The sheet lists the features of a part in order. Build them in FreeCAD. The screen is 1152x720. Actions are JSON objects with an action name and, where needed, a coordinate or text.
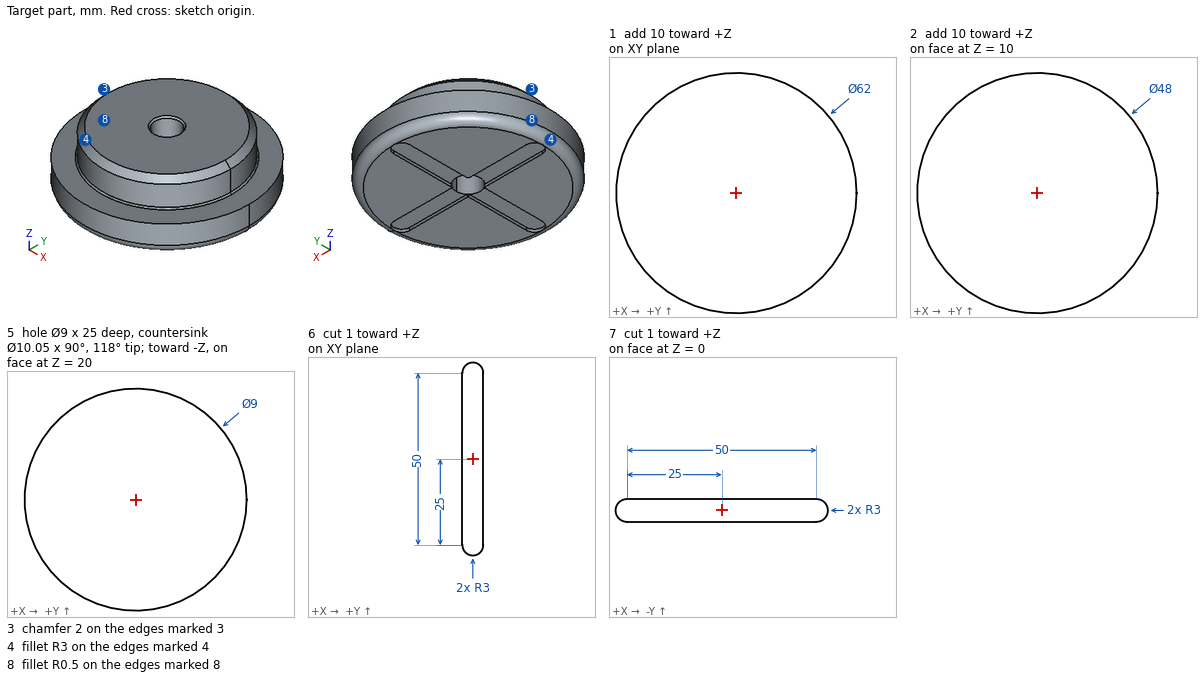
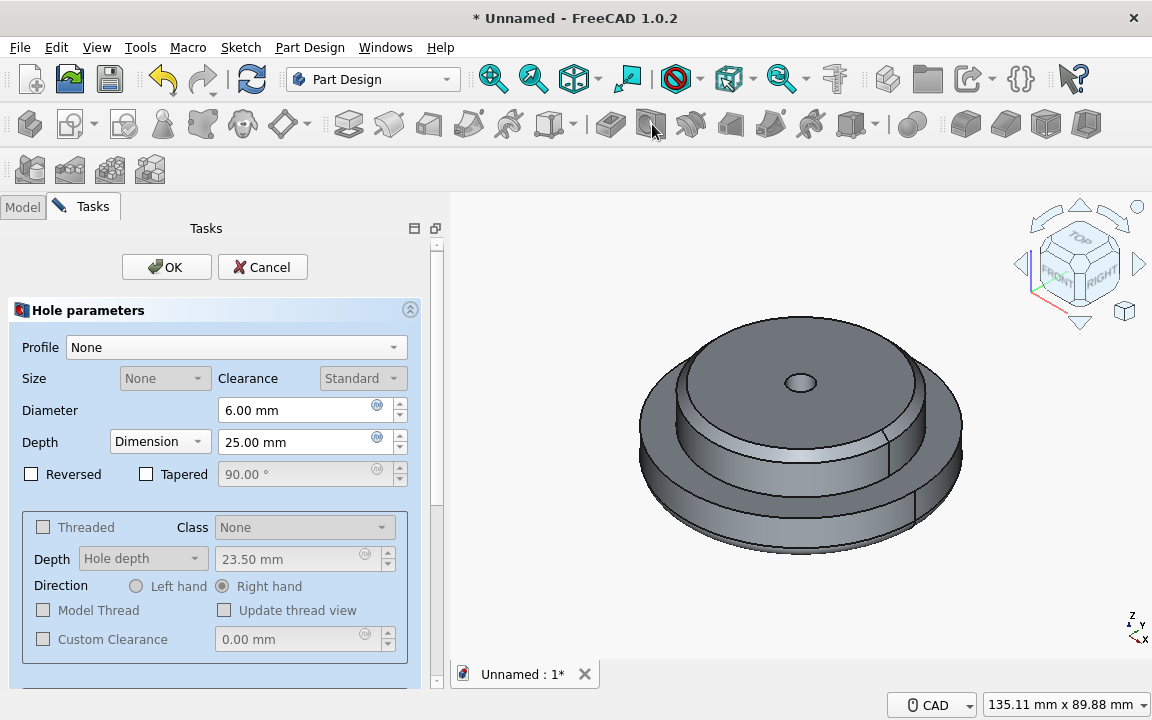
{"action": "triple_click", "coordinate": [305, 410]}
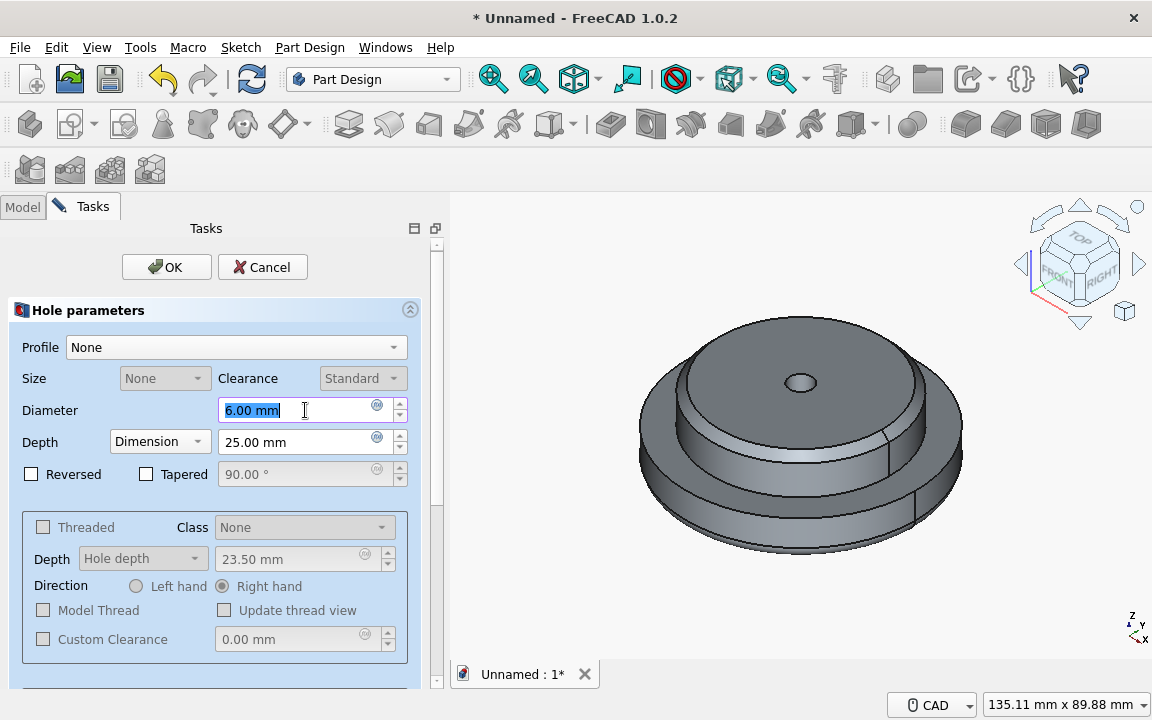
{"action": "type", "text": "9"}
{"action": "key", "text": "Tab"}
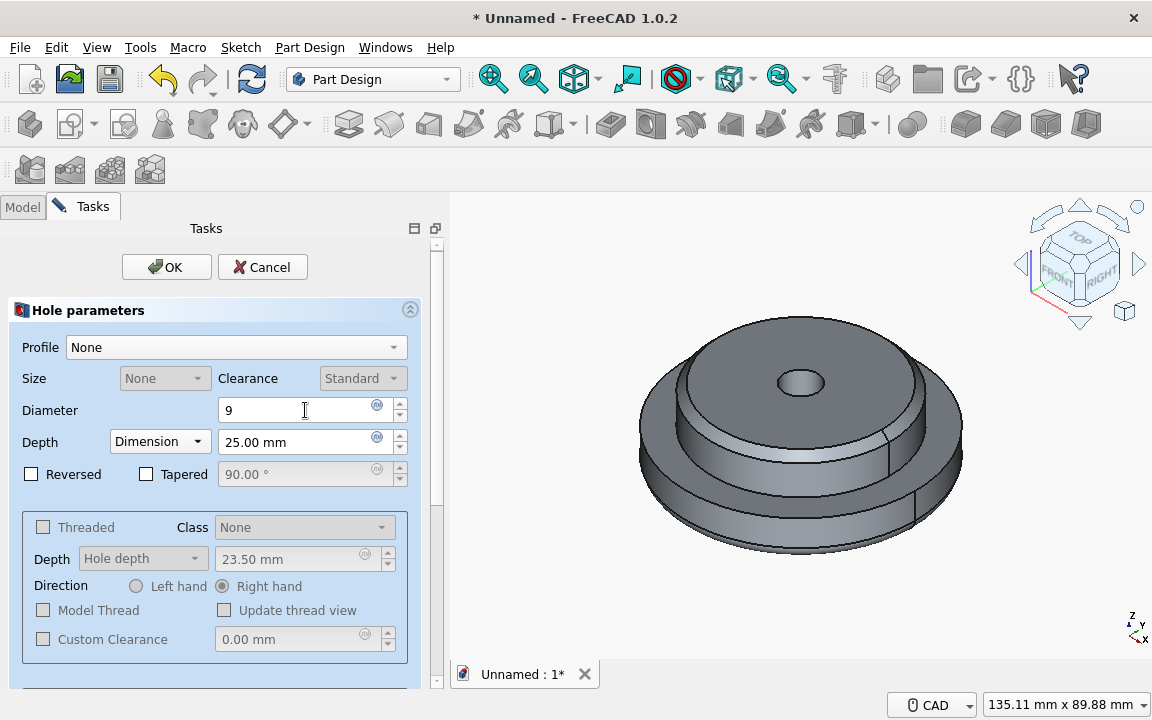
{"action": "triple_click", "coordinate": [305, 442]}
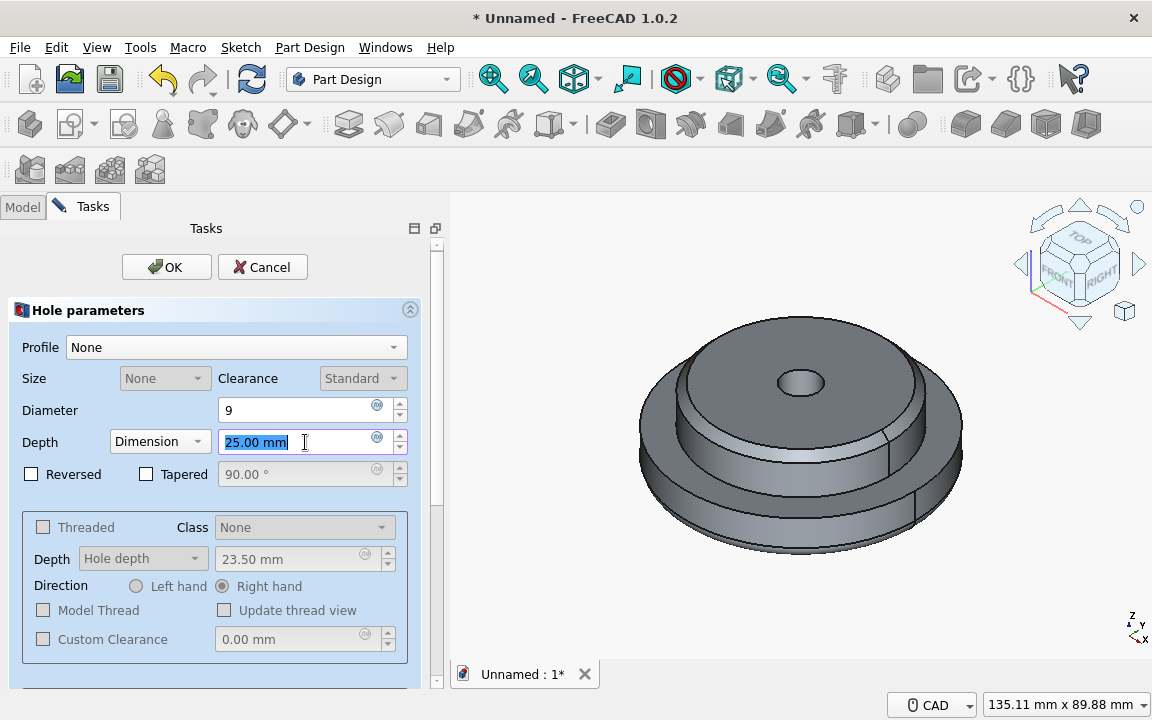
{"action": "type", "text": "25"}
{"action": "key", "text": "Tab"}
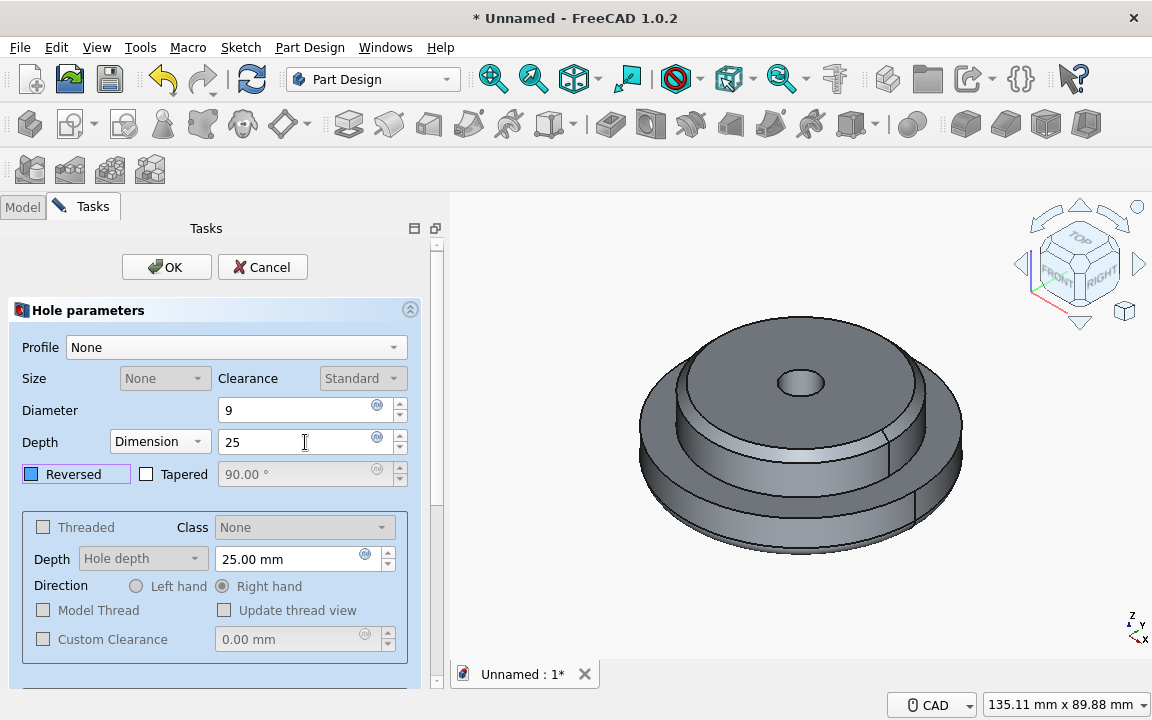
{"action": "scroll", "coordinate": [437, 463], "scroll_direction": "down", "scroll_amount": 2}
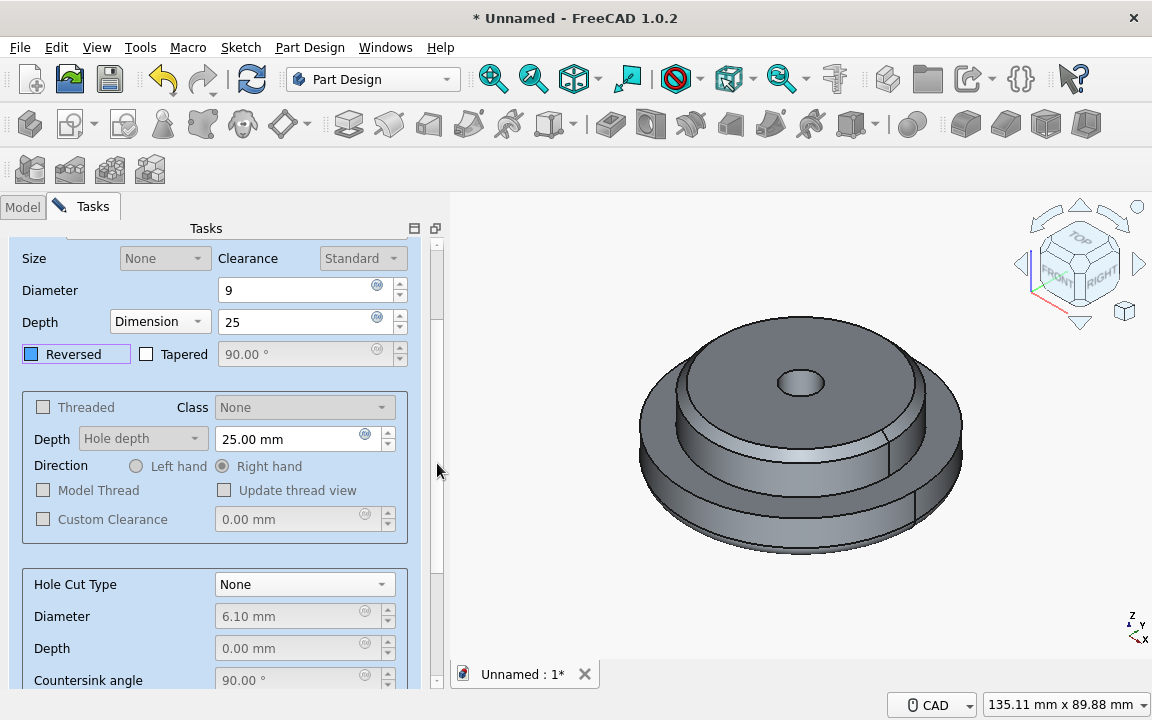
{"action": "left_click", "coordinate": [306, 584]}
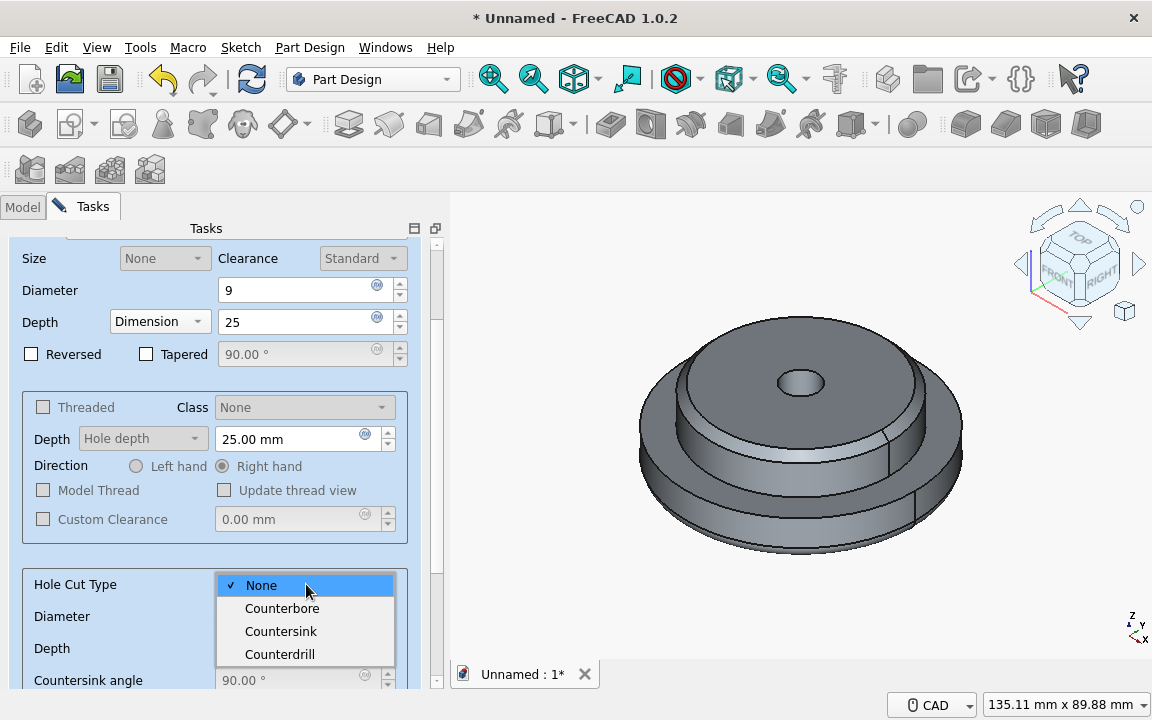
{"action": "left_click", "coordinate": [304, 632]}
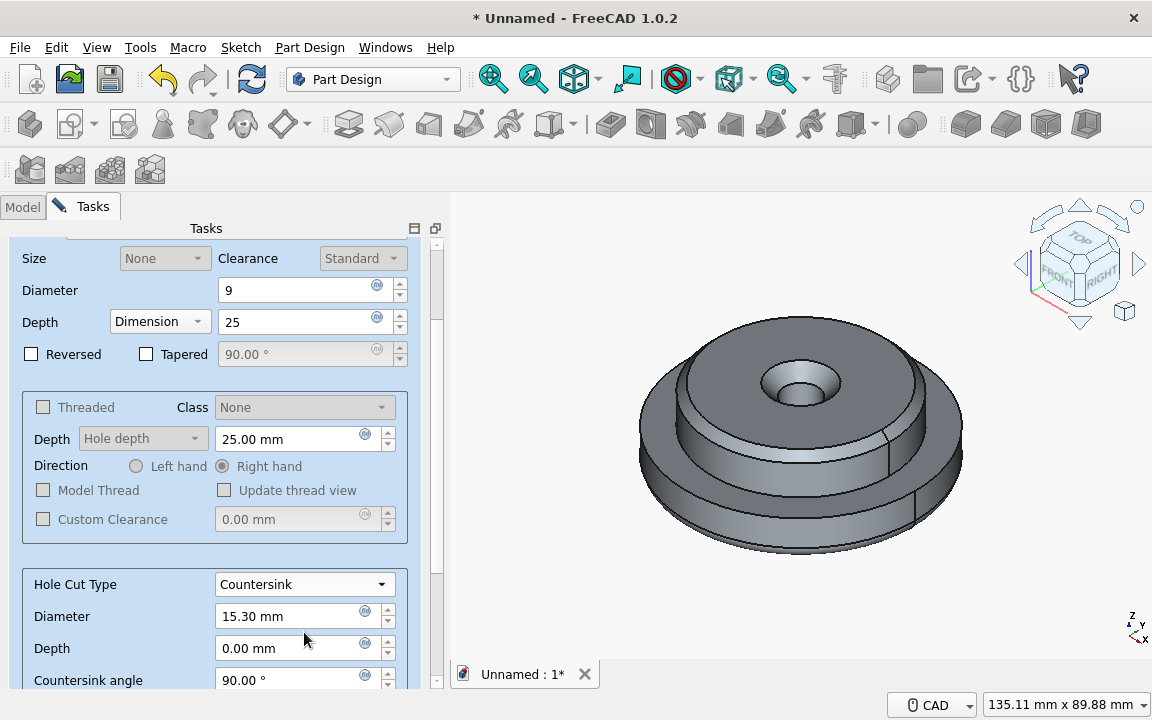
{"action": "triple_click", "coordinate": [298, 616]}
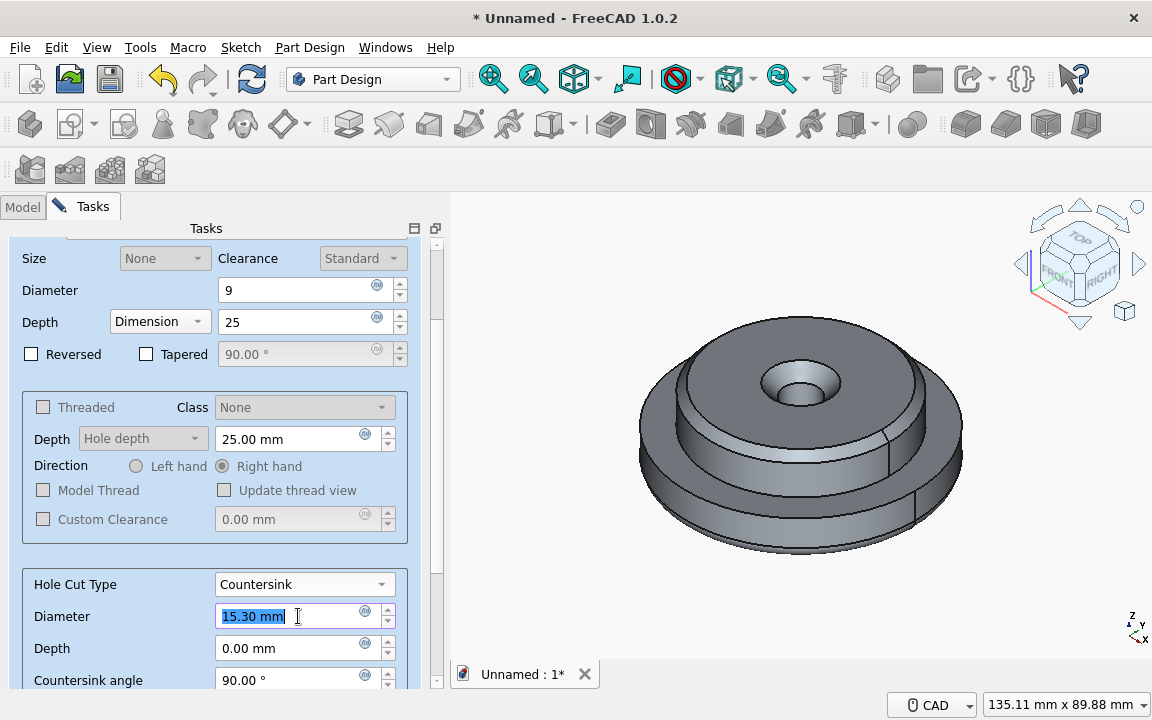
{"action": "type", "text": "10.05"}
{"action": "key", "text": "Tab"}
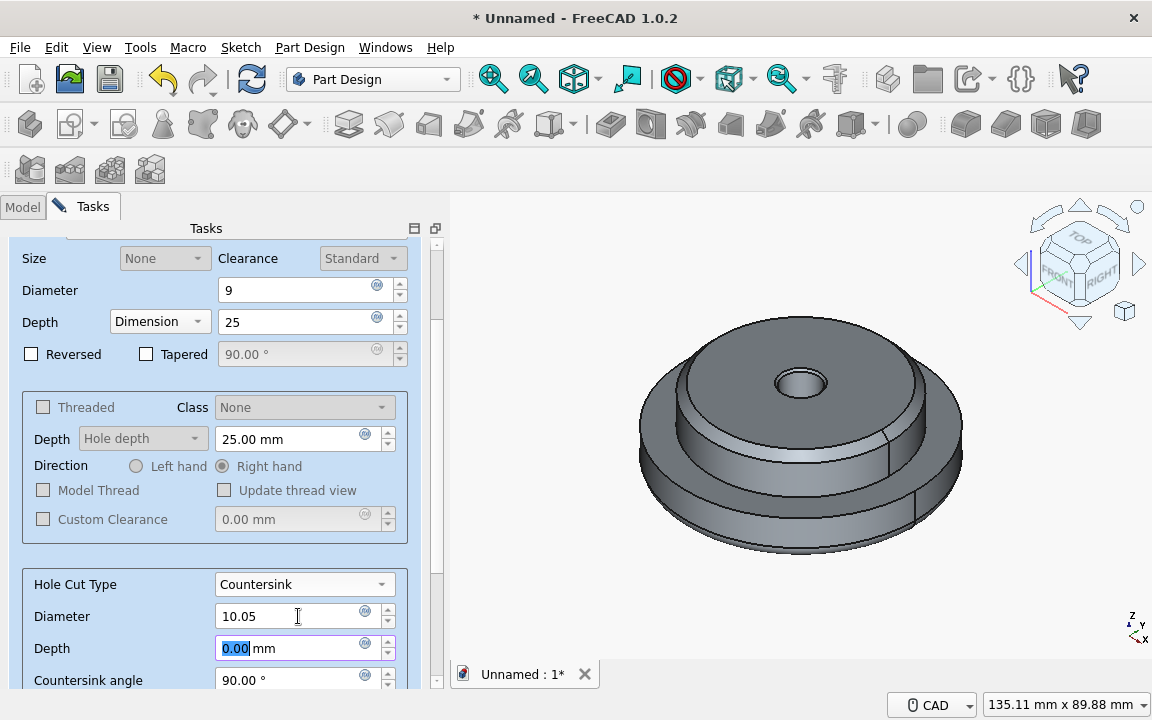
{"action": "scroll", "coordinate": [437, 463], "scroll_direction": "up", "scroll_amount": 3}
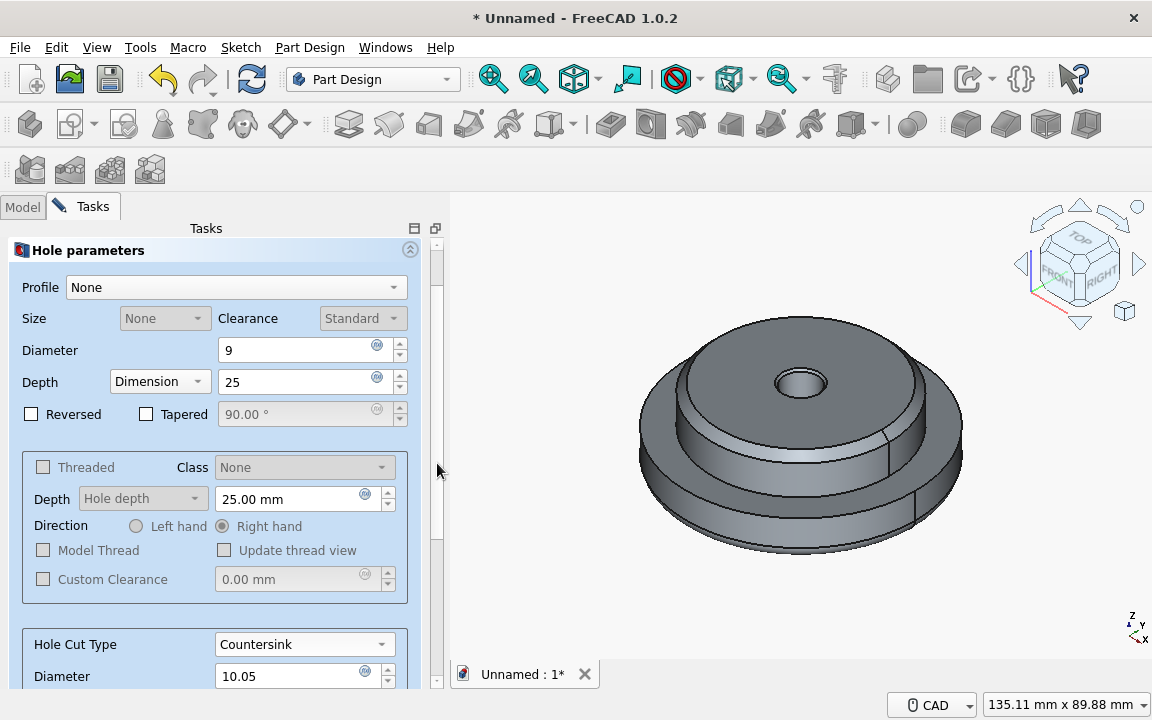
{"action": "left_click", "coordinate": [167, 267]}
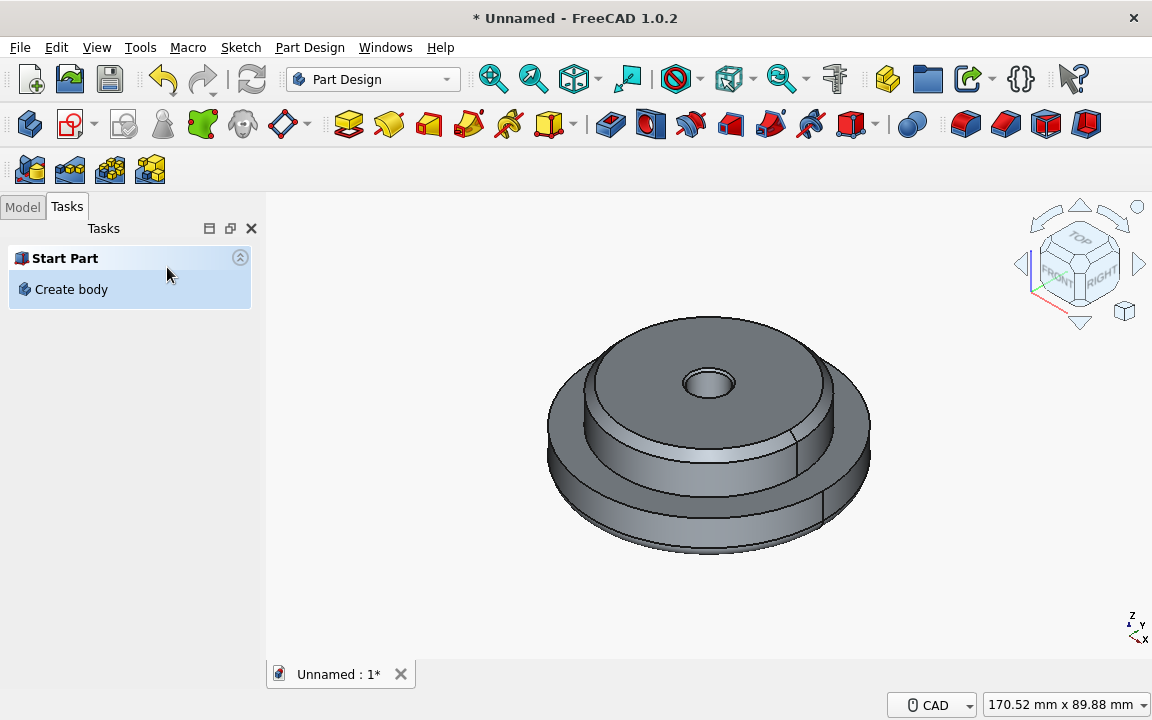
{"action": "left_click", "coordinate": [70, 124]}